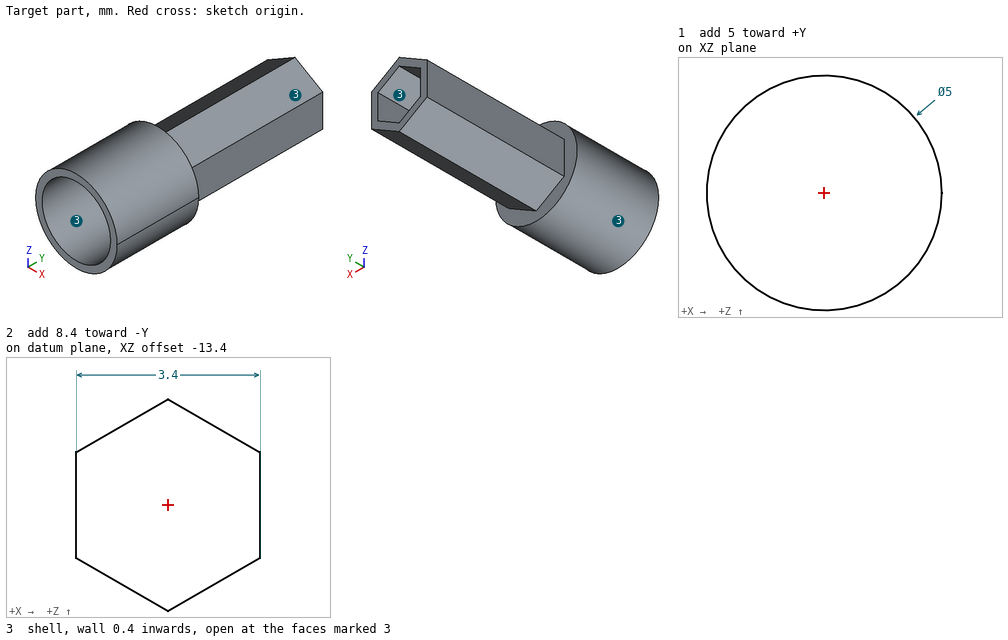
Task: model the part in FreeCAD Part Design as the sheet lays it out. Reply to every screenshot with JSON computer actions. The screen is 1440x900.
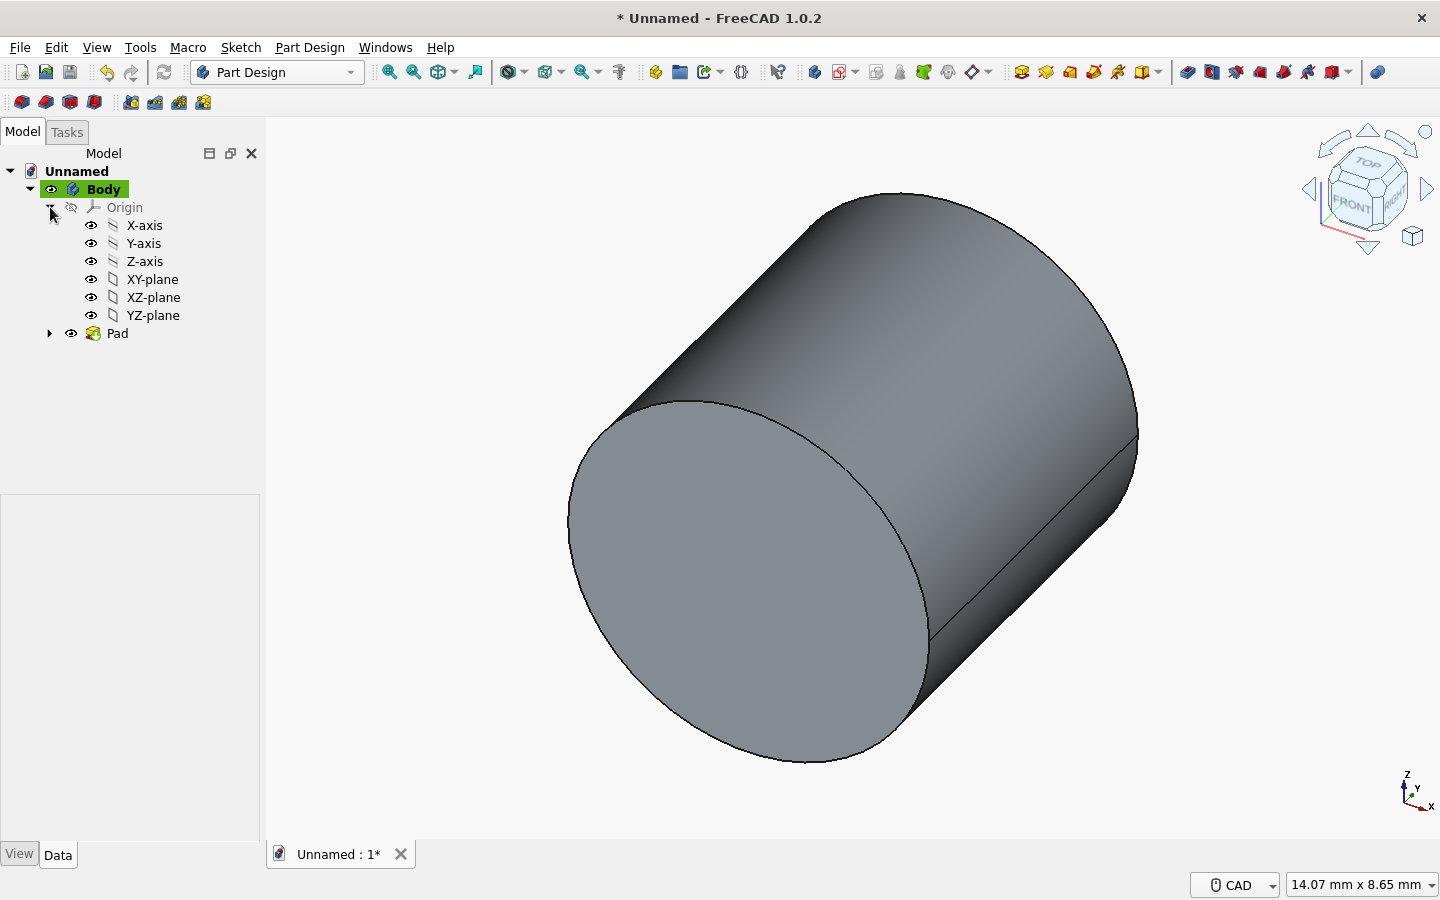
{"action": "left_click", "coordinate": [136, 297]}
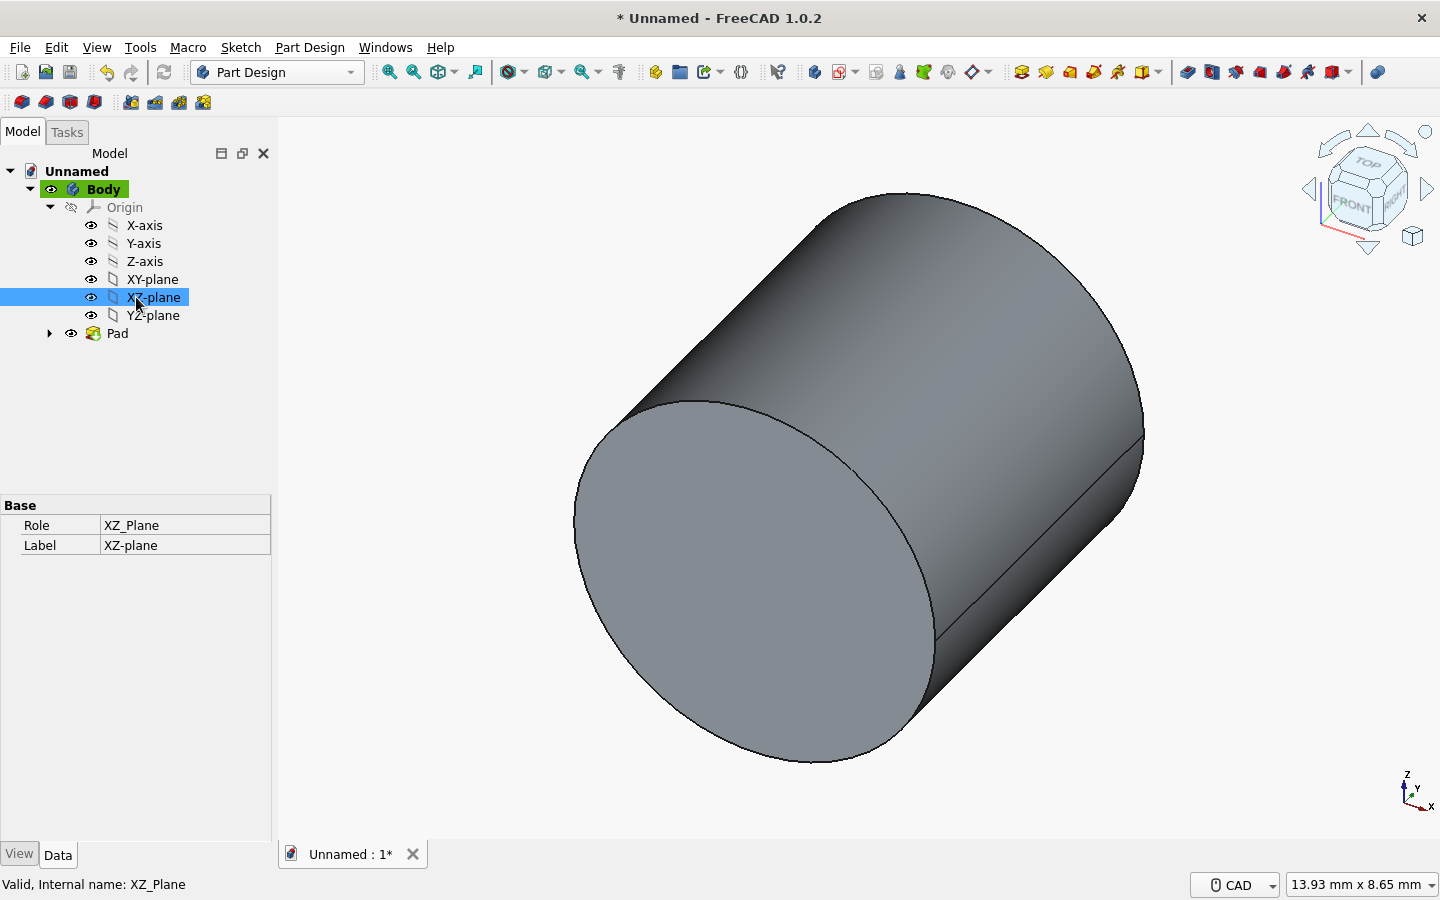
{"action": "left_click", "coordinate": [972, 72]}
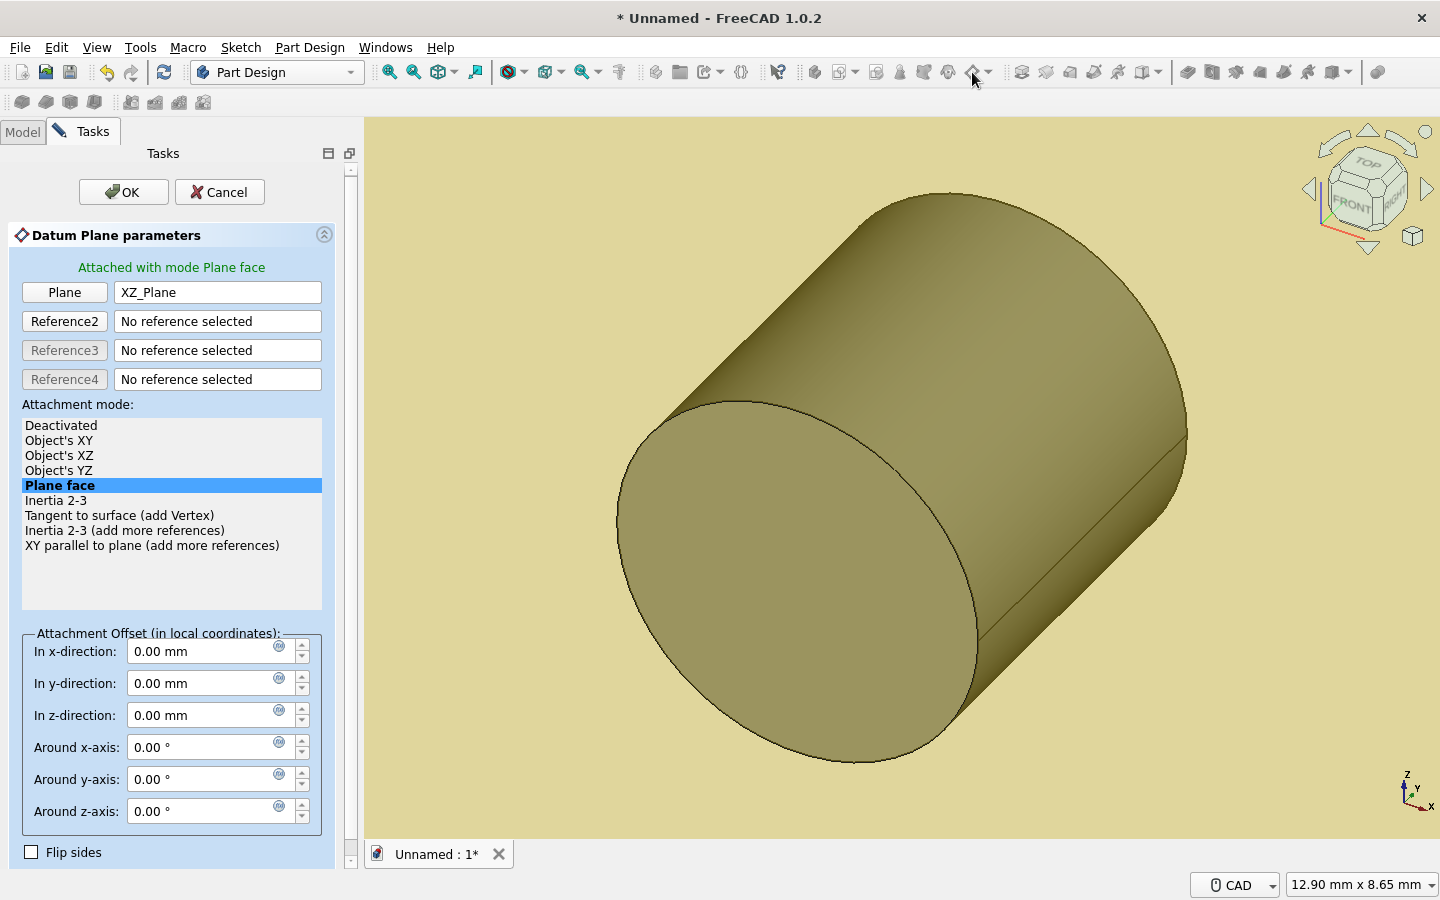
{"action": "triple_click", "coordinate": [210, 715]}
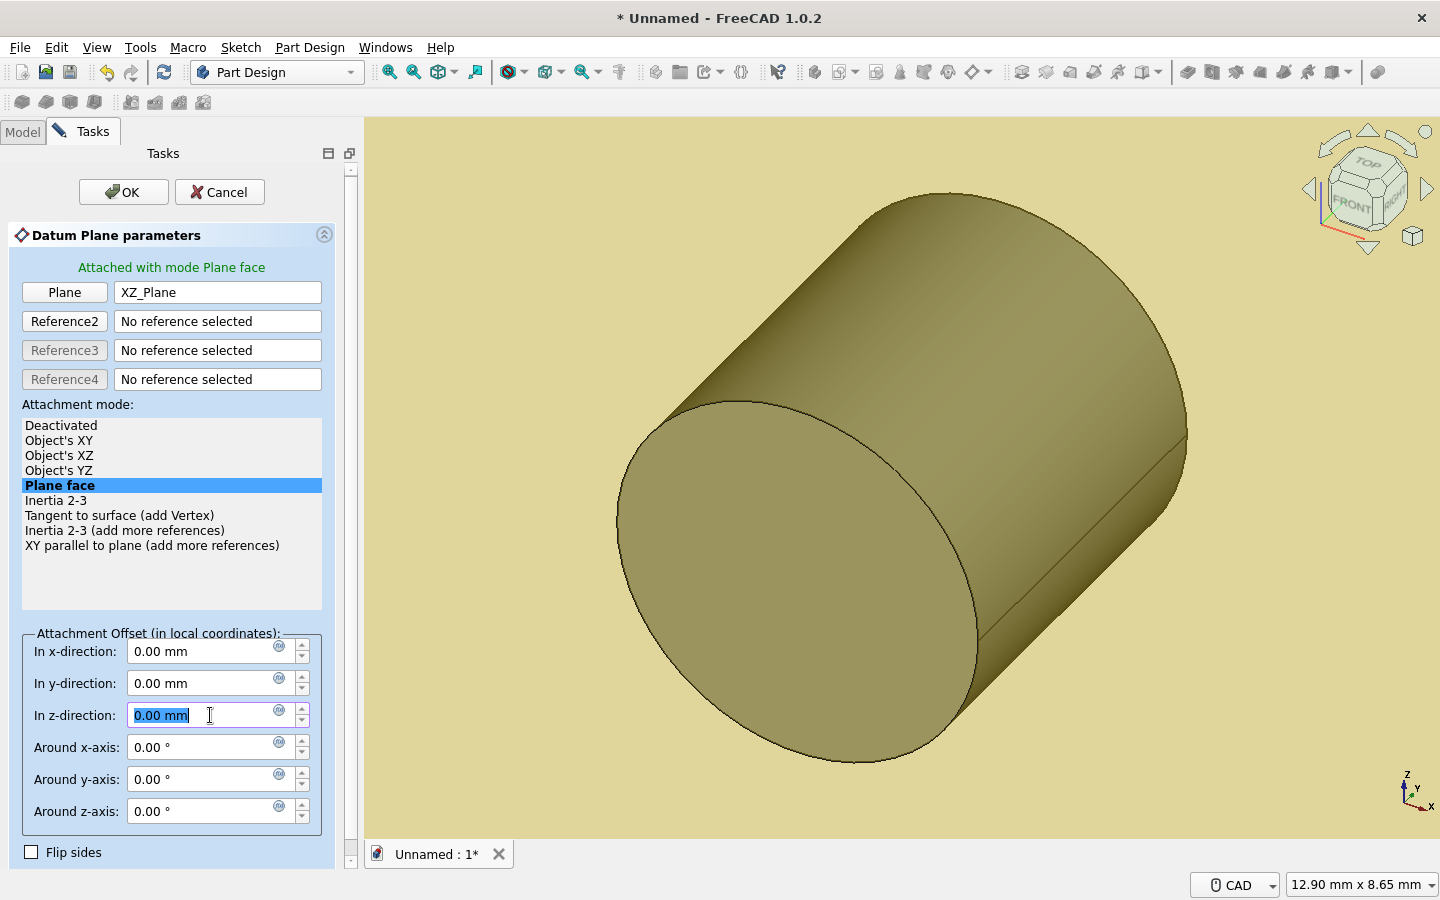
{"action": "type", "text": "-13.4"}
{"action": "key", "text": "Tab"}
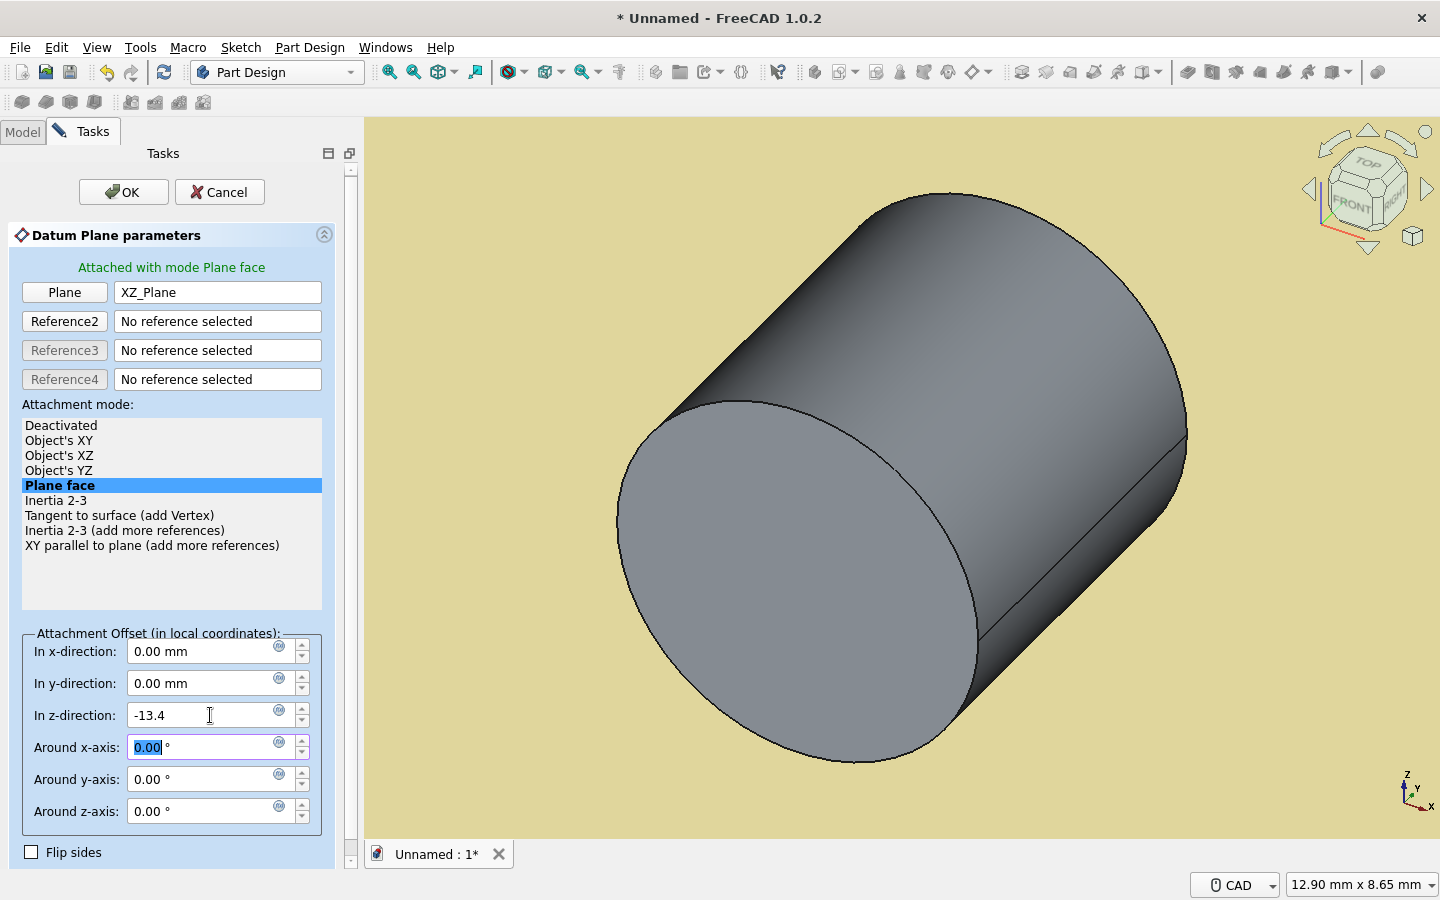
{"action": "left_click", "coordinate": [124, 192]}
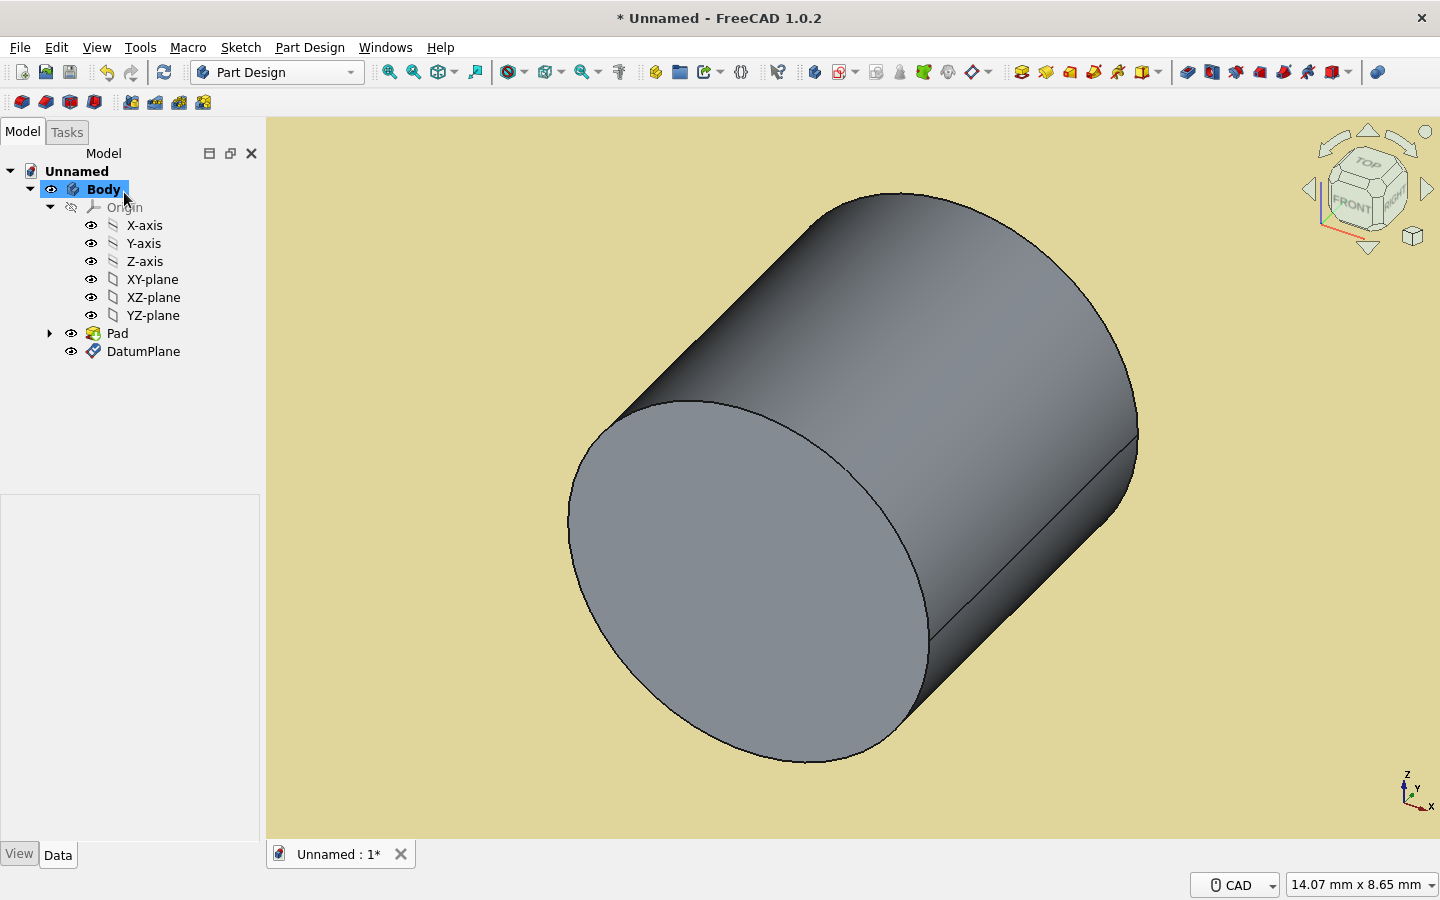
{"action": "left_click", "coordinate": [116, 351]}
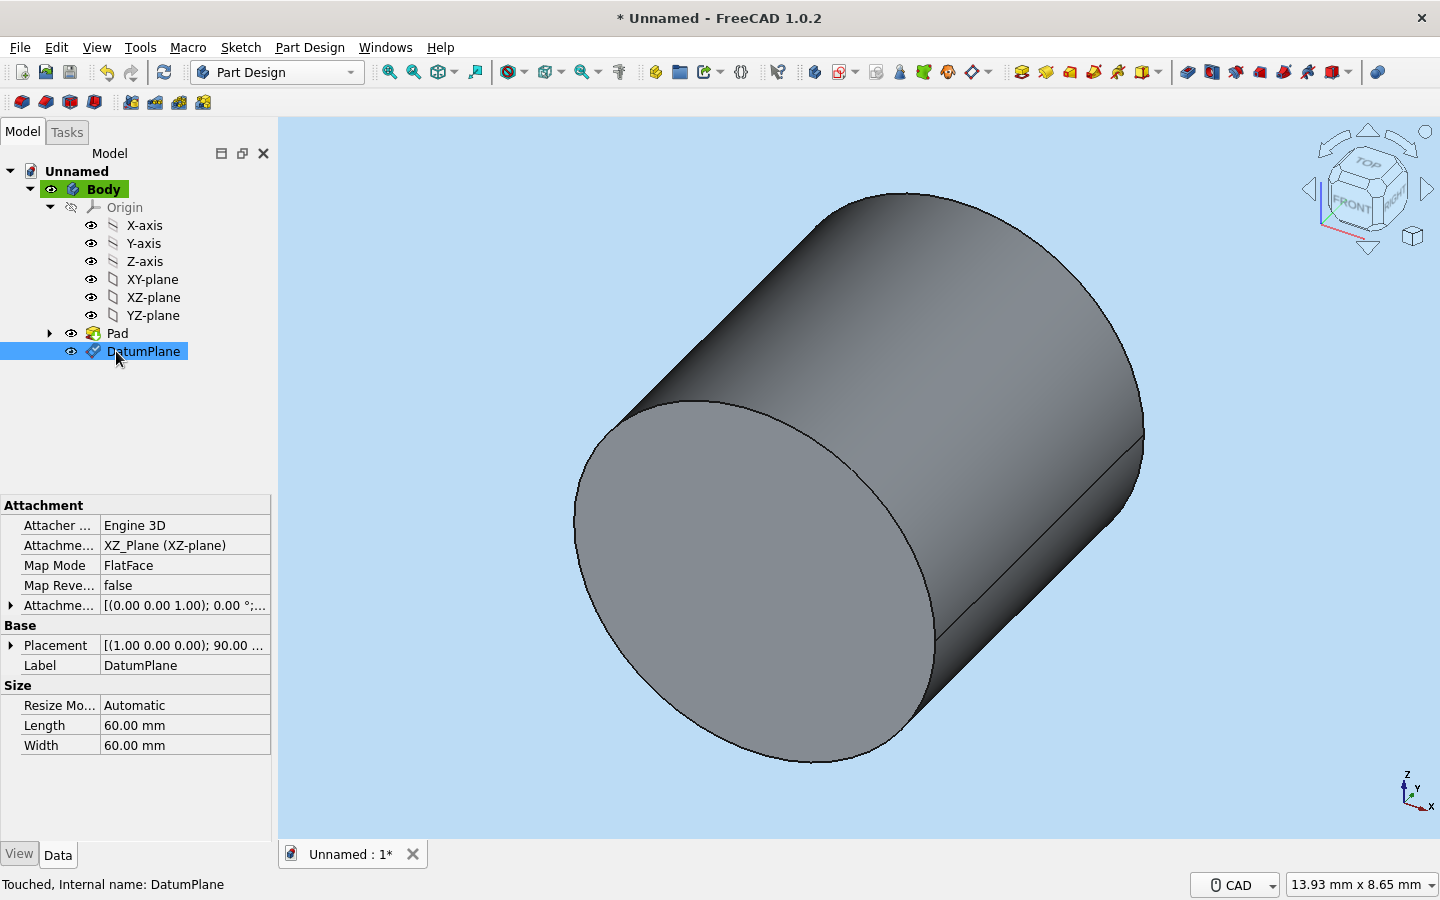
{"action": "left_click", "coordinate": [840, 72]}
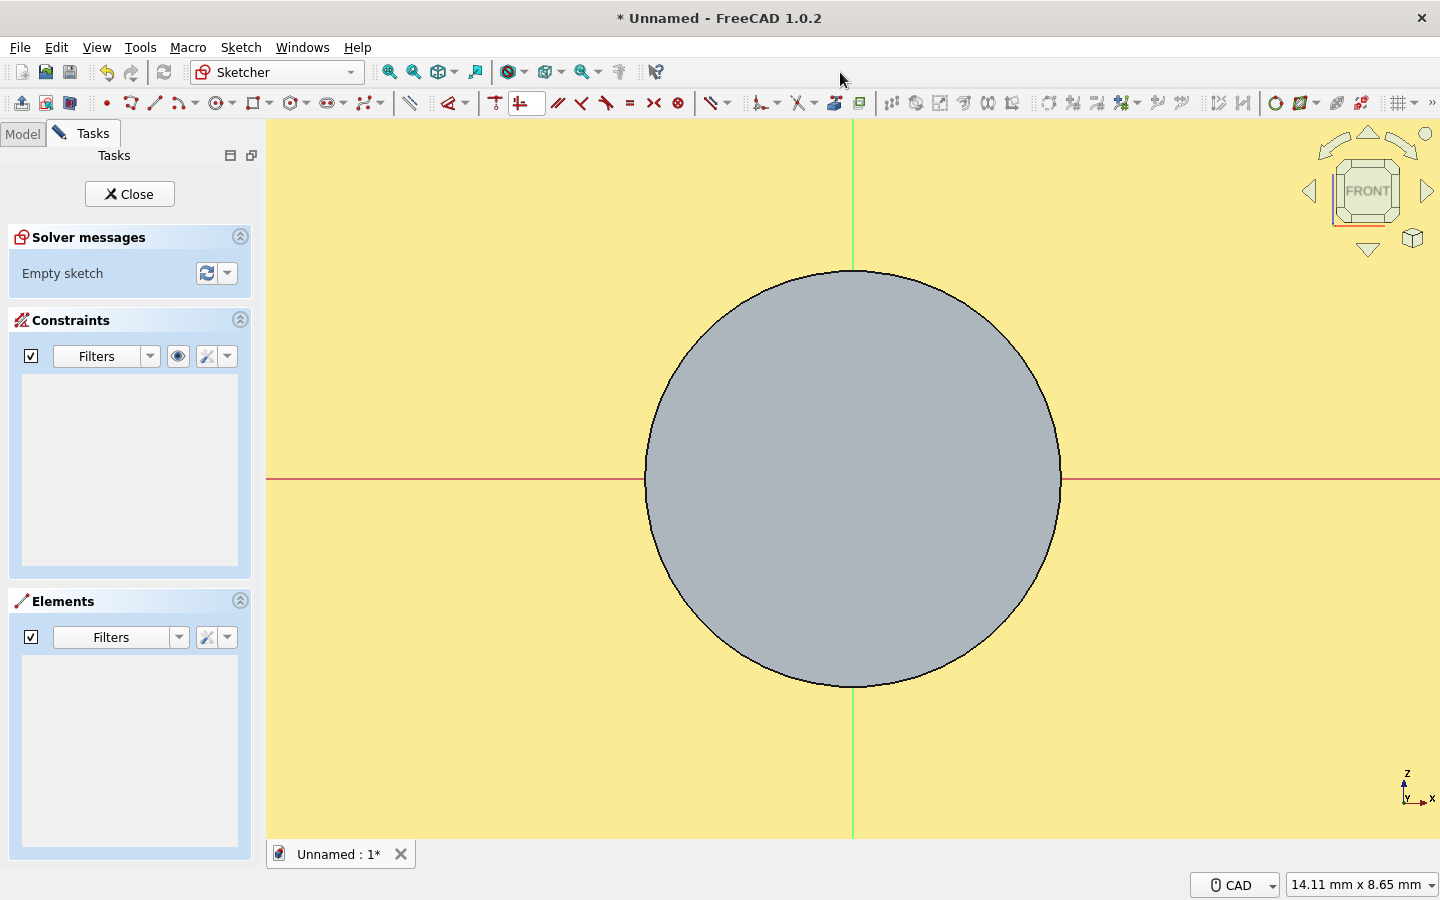
{"action": "left_click", "coordinate": [70, 104]}